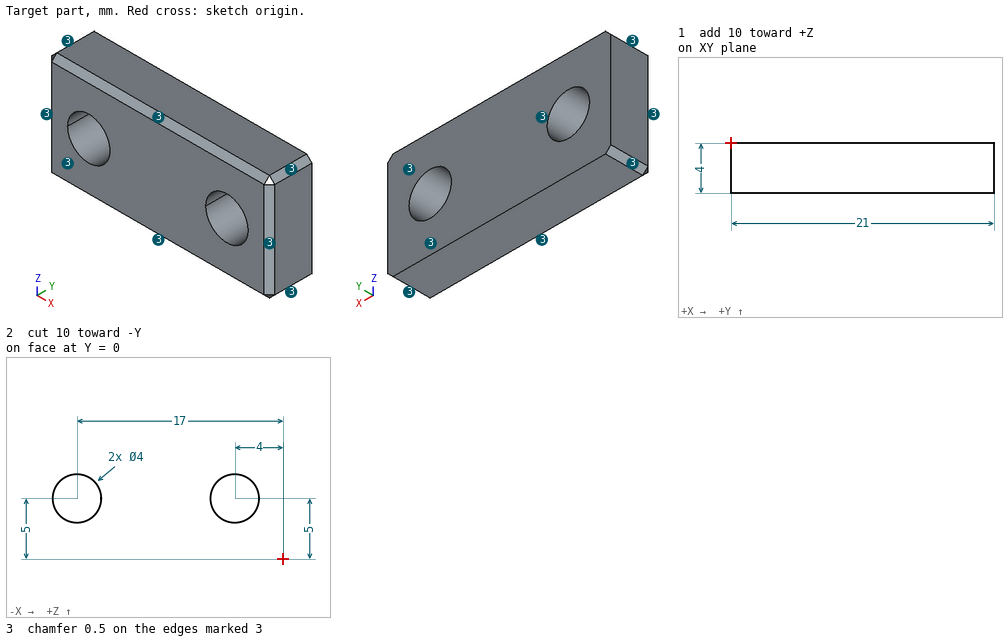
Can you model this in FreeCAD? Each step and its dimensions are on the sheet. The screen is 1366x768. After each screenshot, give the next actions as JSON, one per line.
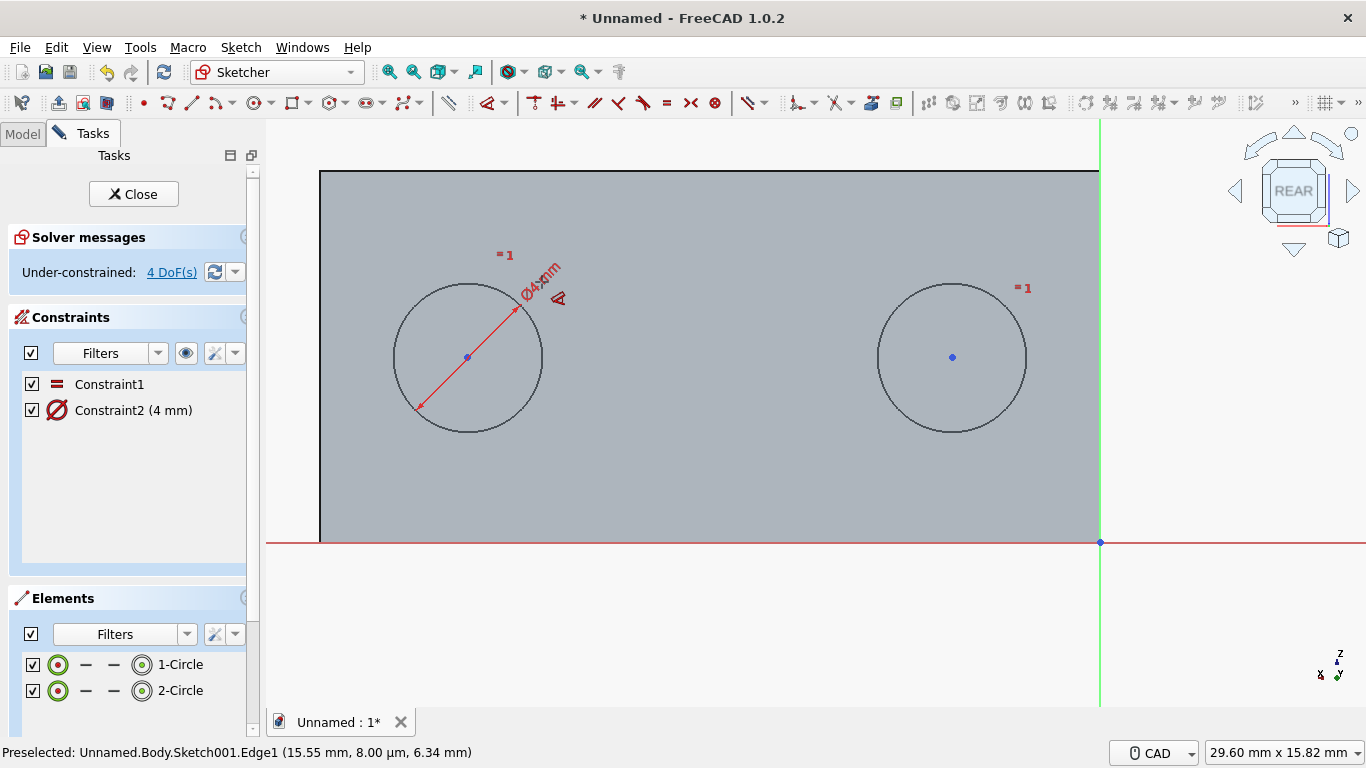
{"action": "left_click", "coordinate": [468, 358]}
{"action": "left_click", "coordinate": [1134, 450]}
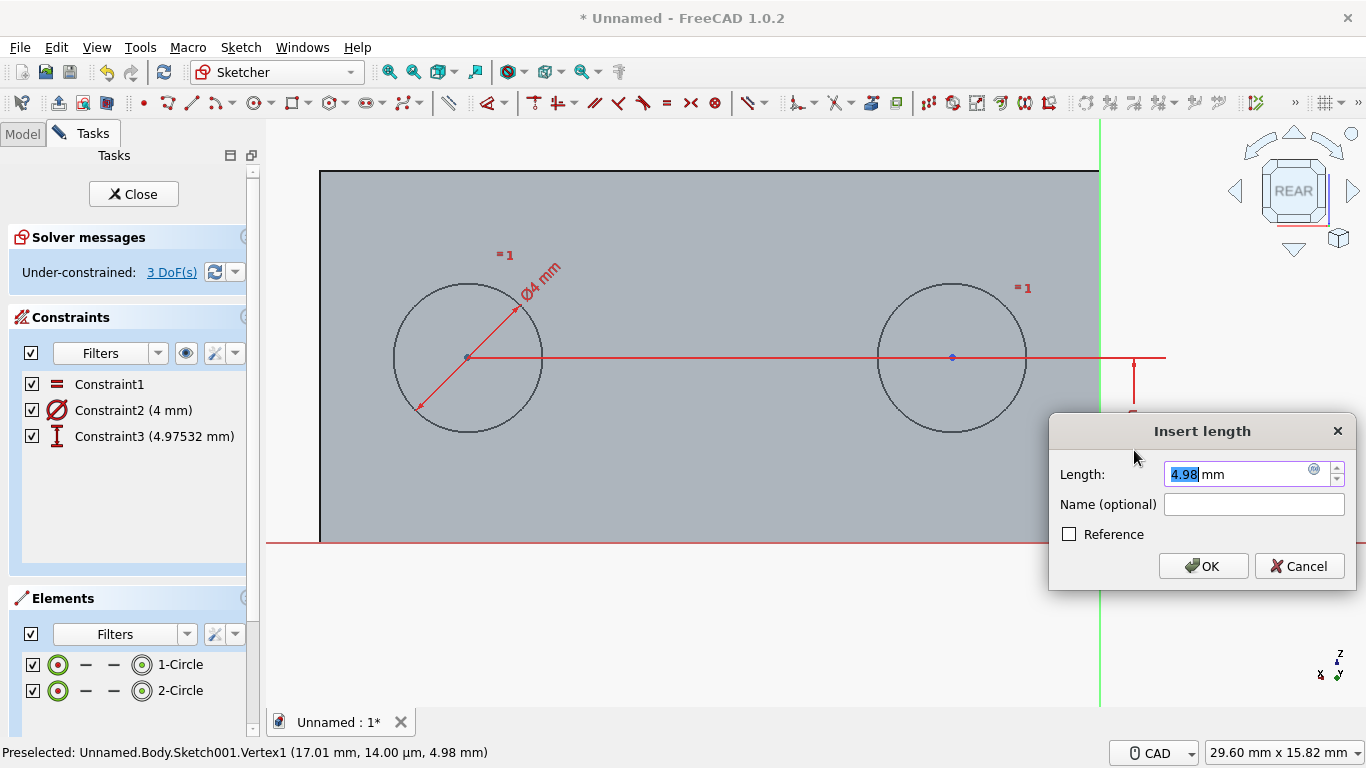
{"action": "type", "text": "5"}
{"action": "key", "text": "Return"}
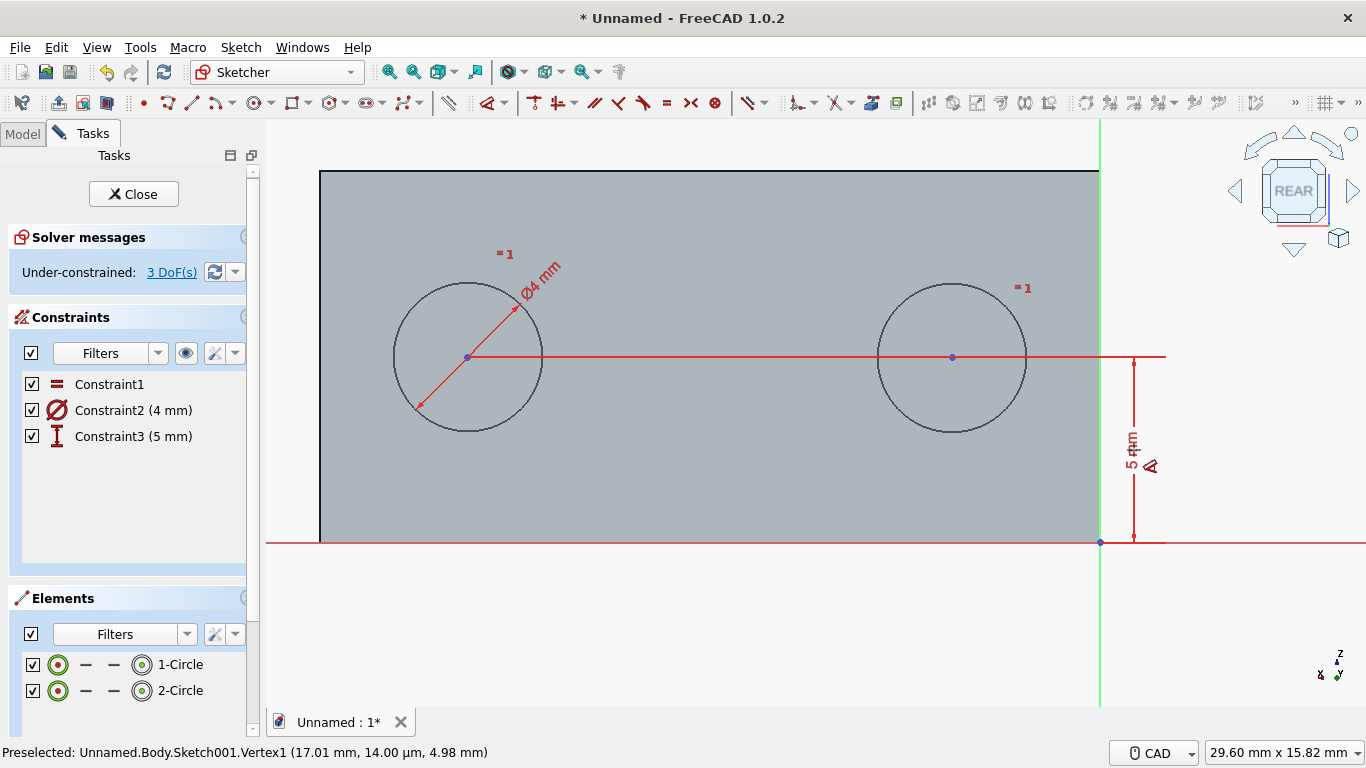
{"action": "left_click", "coordinate": [952, 358]}
{"action": "left_click", "coordinate": [1026, 577]}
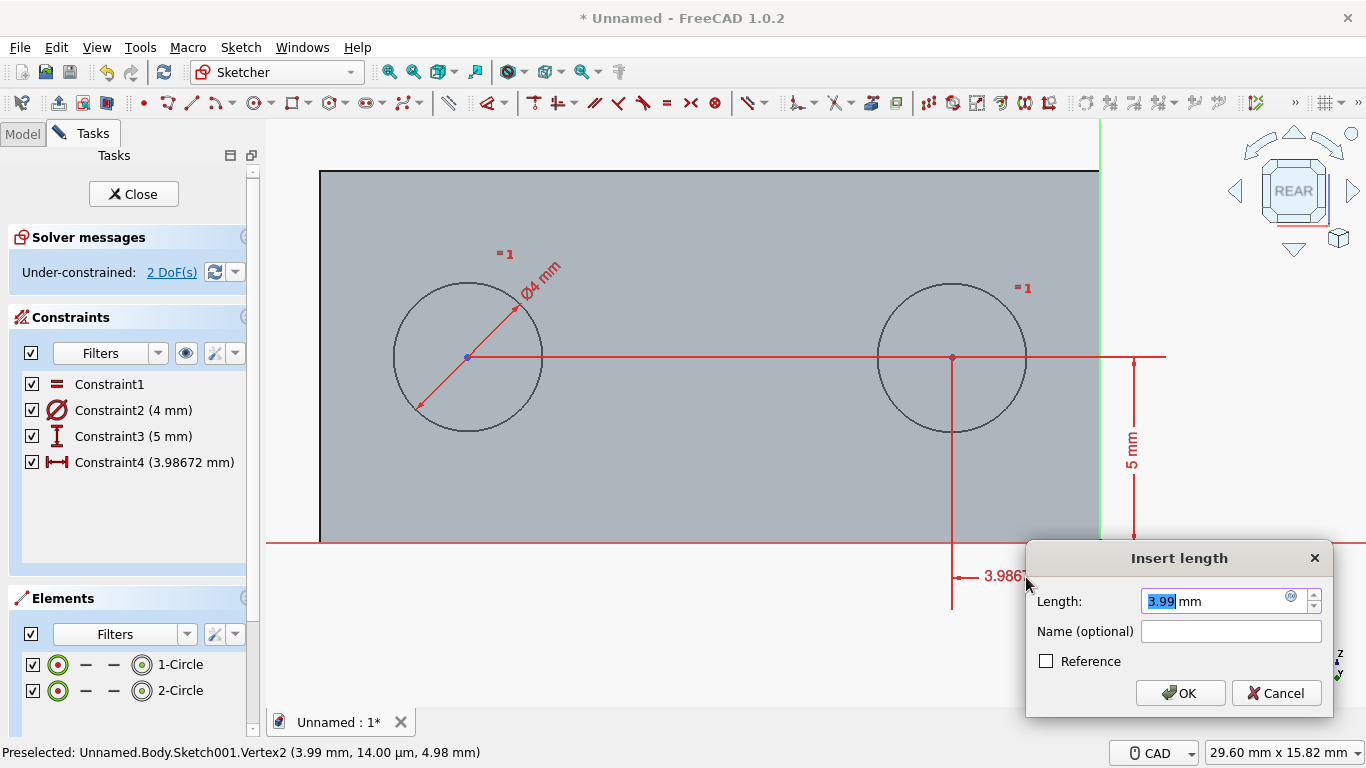
{"action": "type", "text": "4"}
{"action": "key", "text": "Return"}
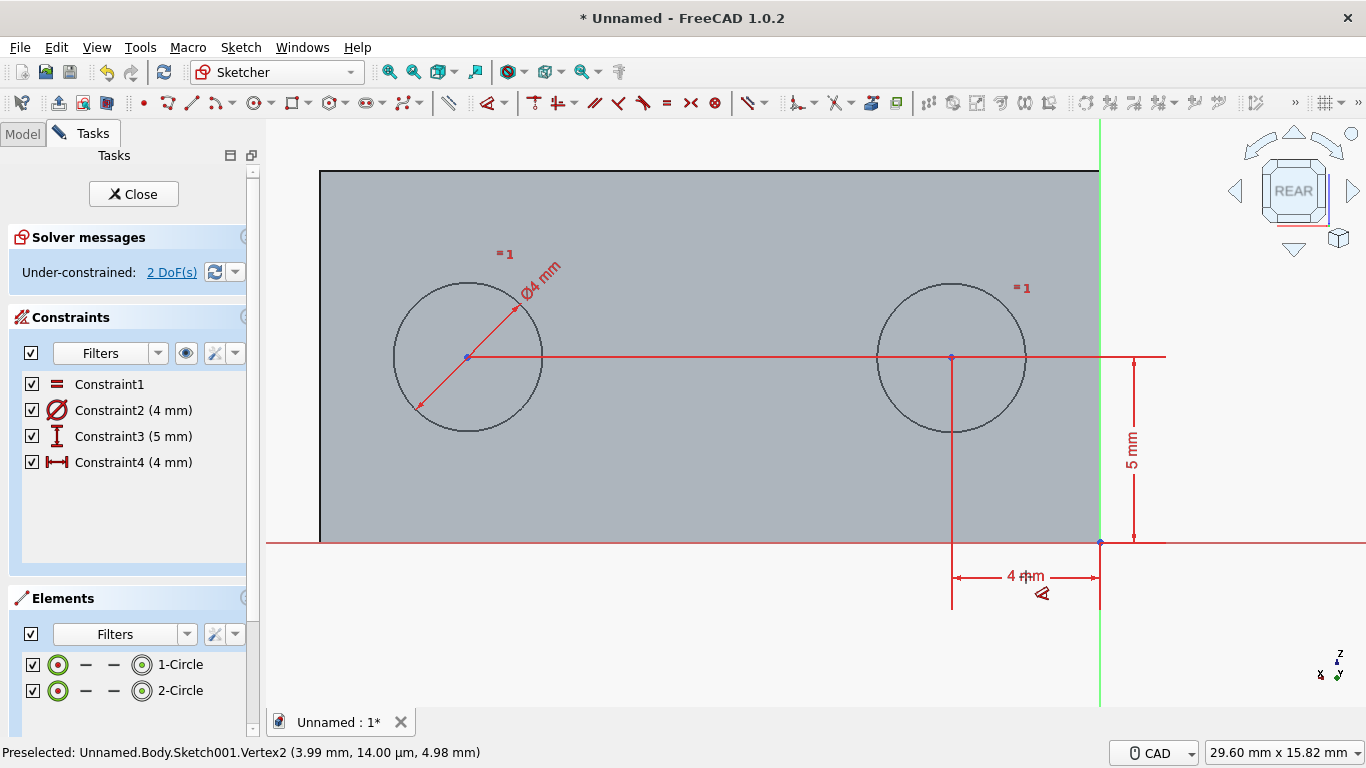
{"action": "left_click", "coordinate": [952, 358]}
{"action": "left_click", "coordinate": [1134, 408]}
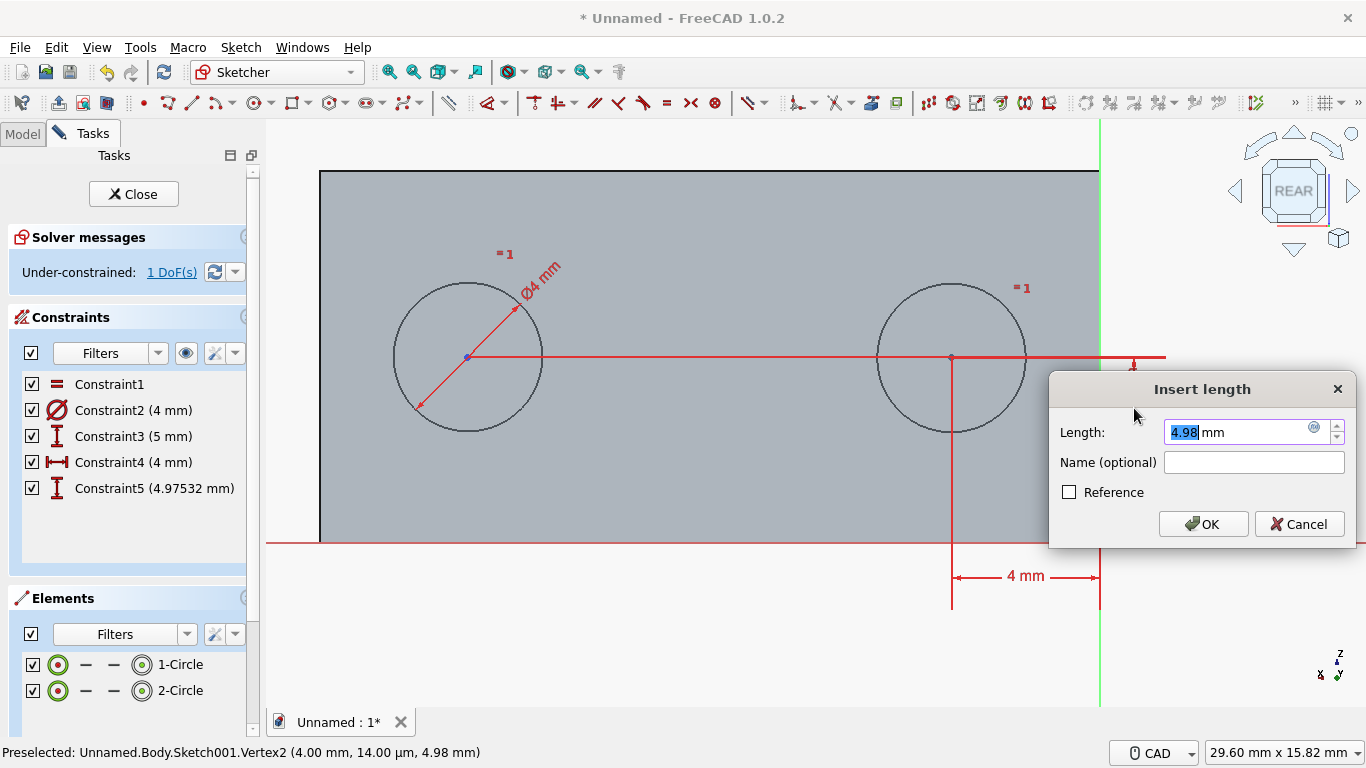
{"action": "type", "text": "5"}
{"action": "key", "text": "Return"}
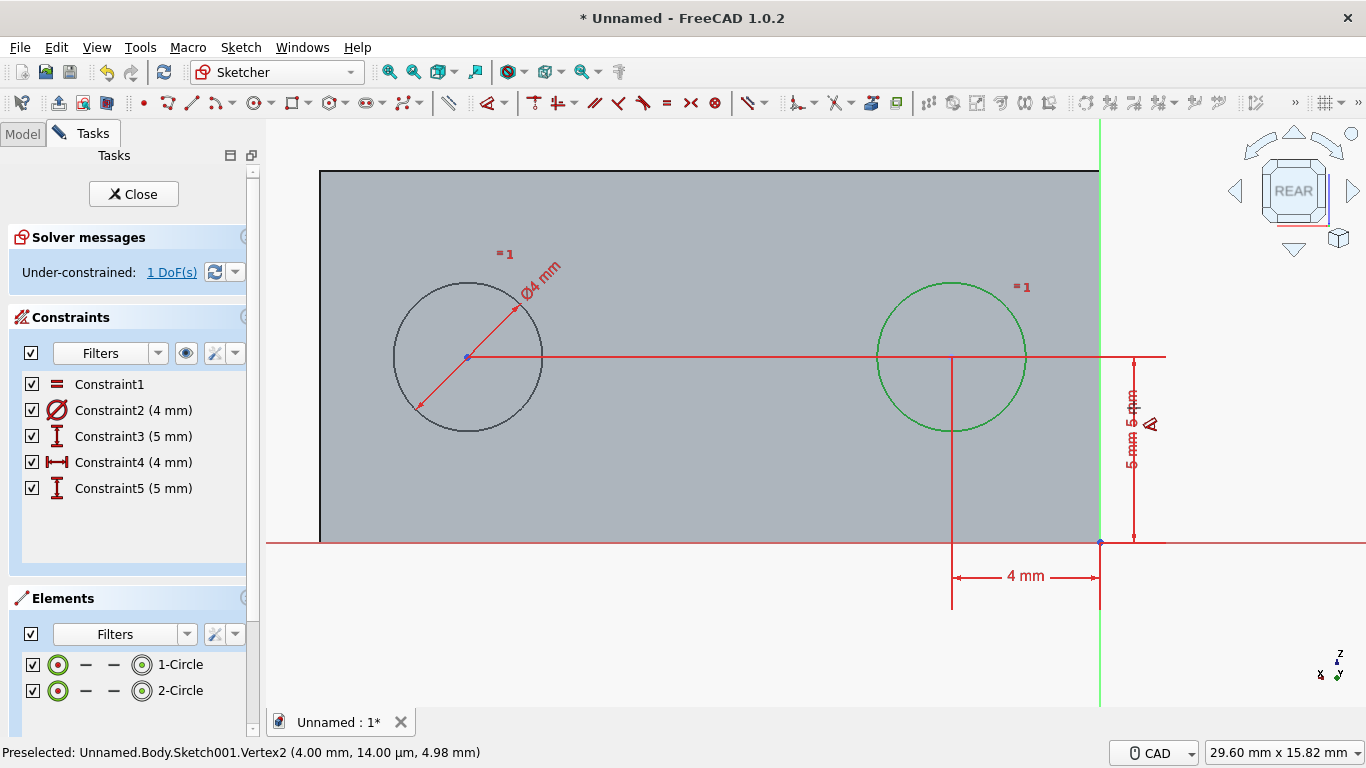
{"action": "left_click", "coordinate": [468, 357]}
{"action": "left_click", "coordinate": [784, 577]}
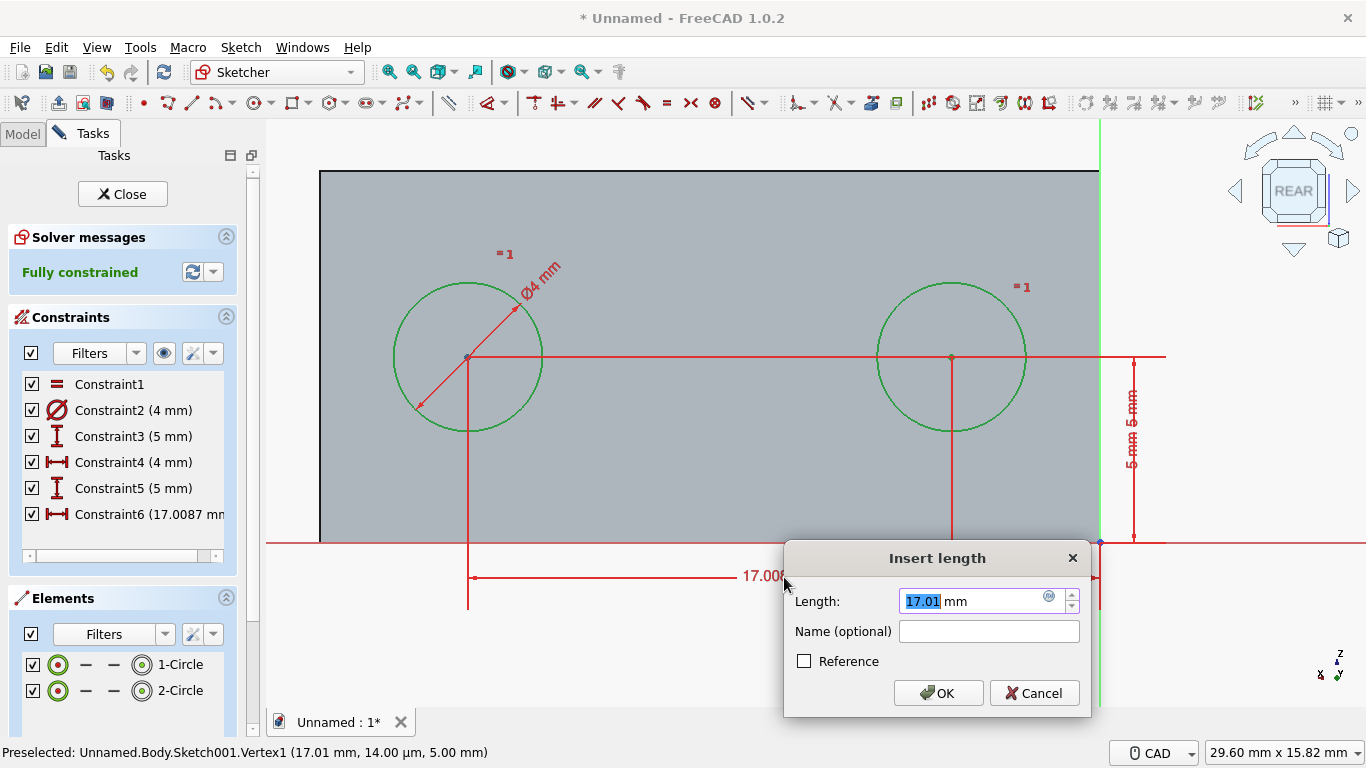
{"action": "type", "text": "17"}
{"action": "key", "text": "Return"}
{"action": "key", "text": "Escape"}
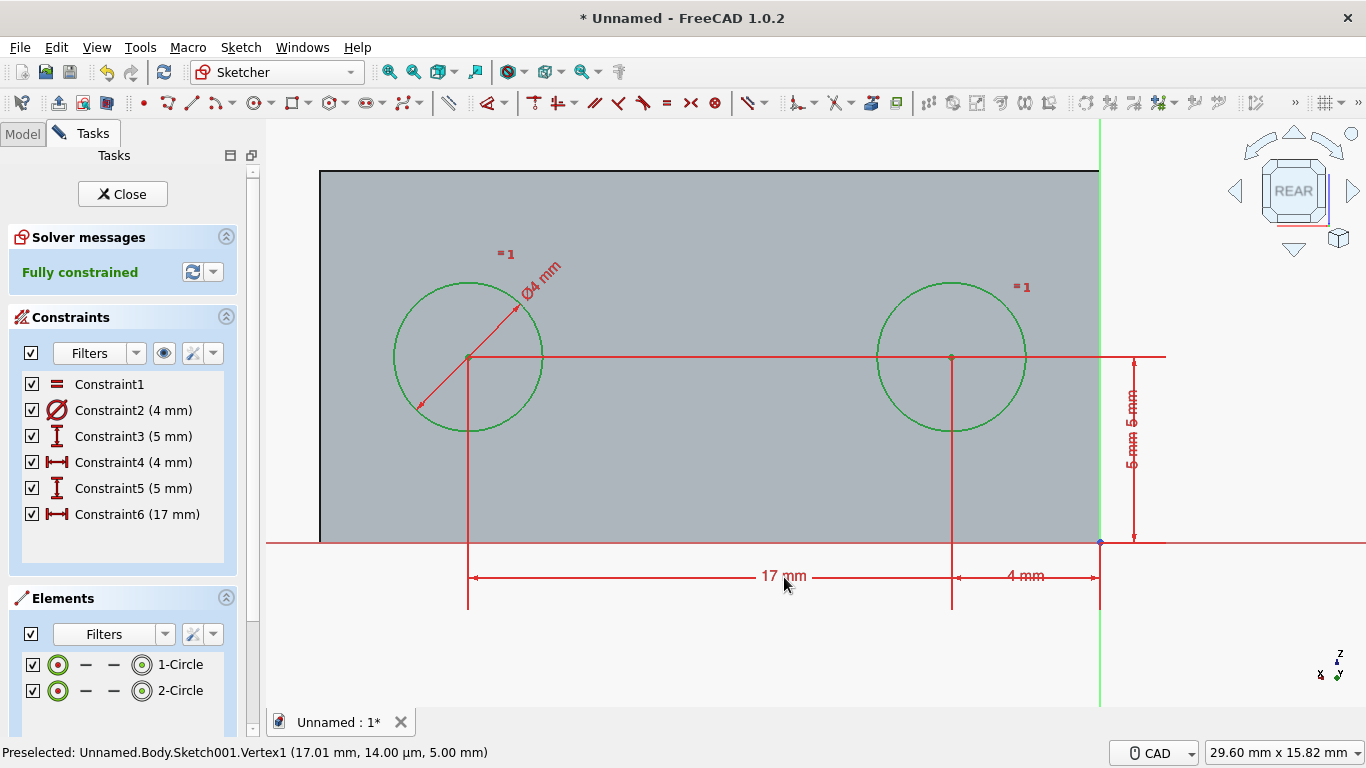
{"action": "left_click", "coordinate": [123, 194]}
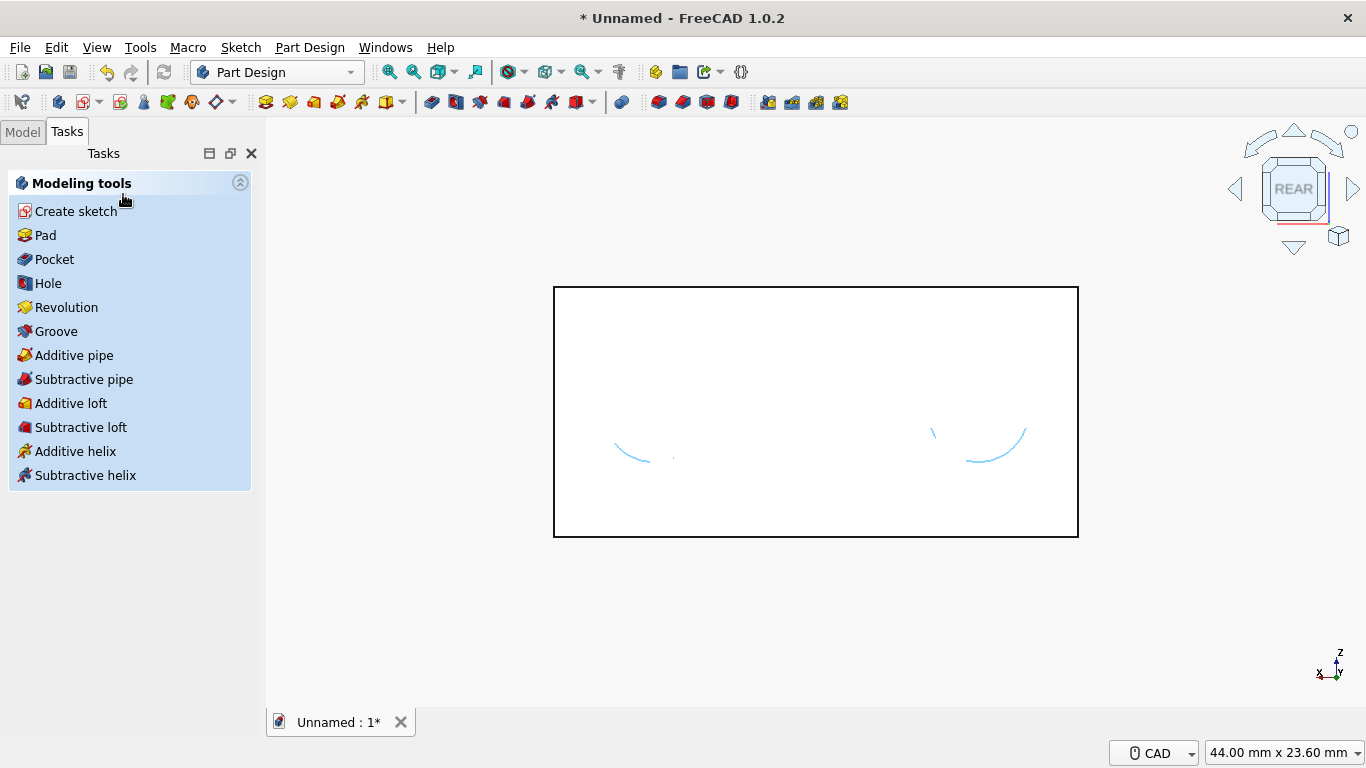
{"action": "left_click", "coordinate": [432, 102]}